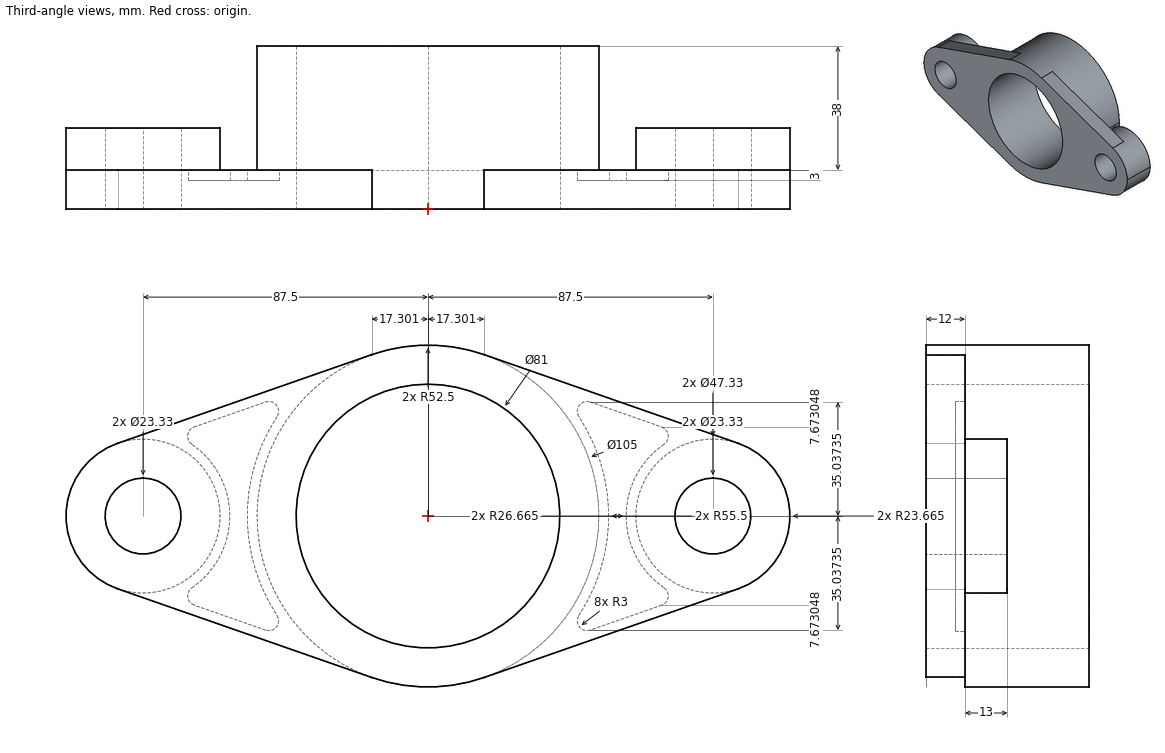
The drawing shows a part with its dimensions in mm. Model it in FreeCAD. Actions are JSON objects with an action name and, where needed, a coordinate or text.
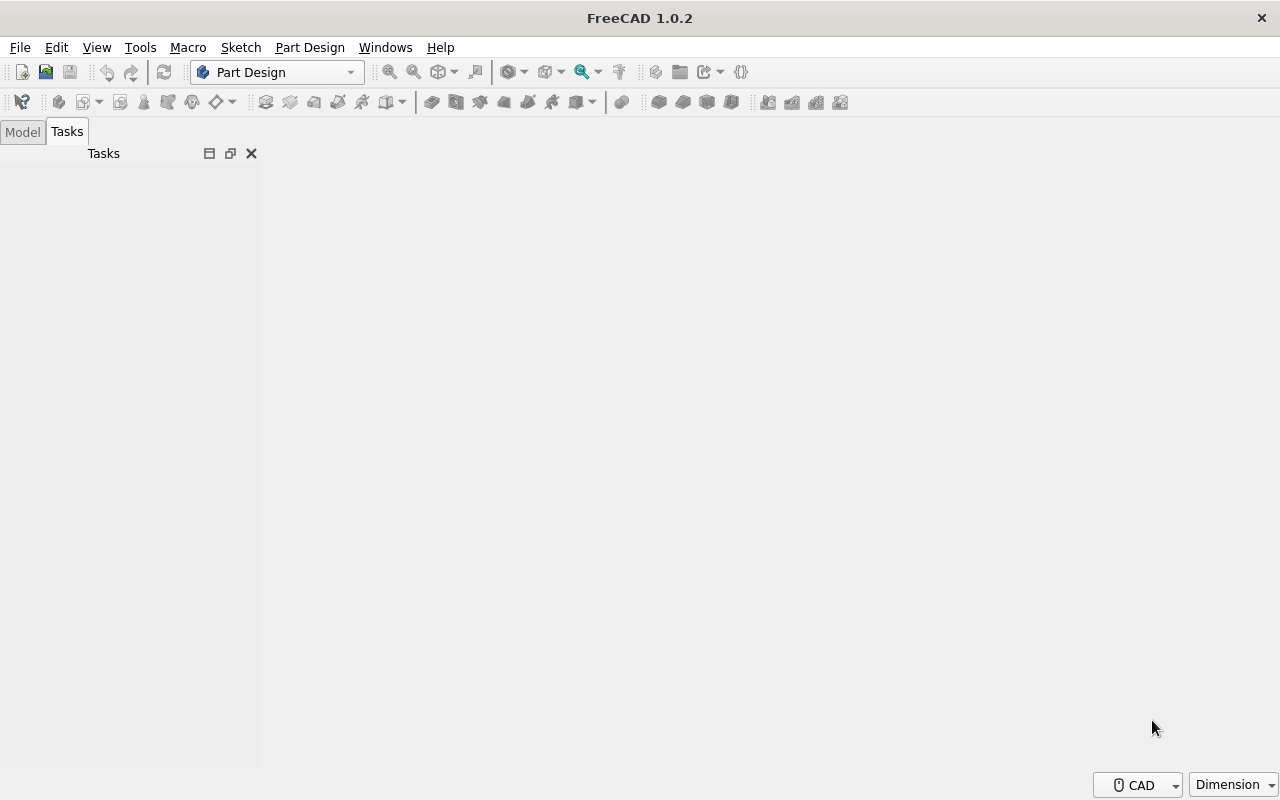
{"action": "left_click", "coordinate": [22, 72]}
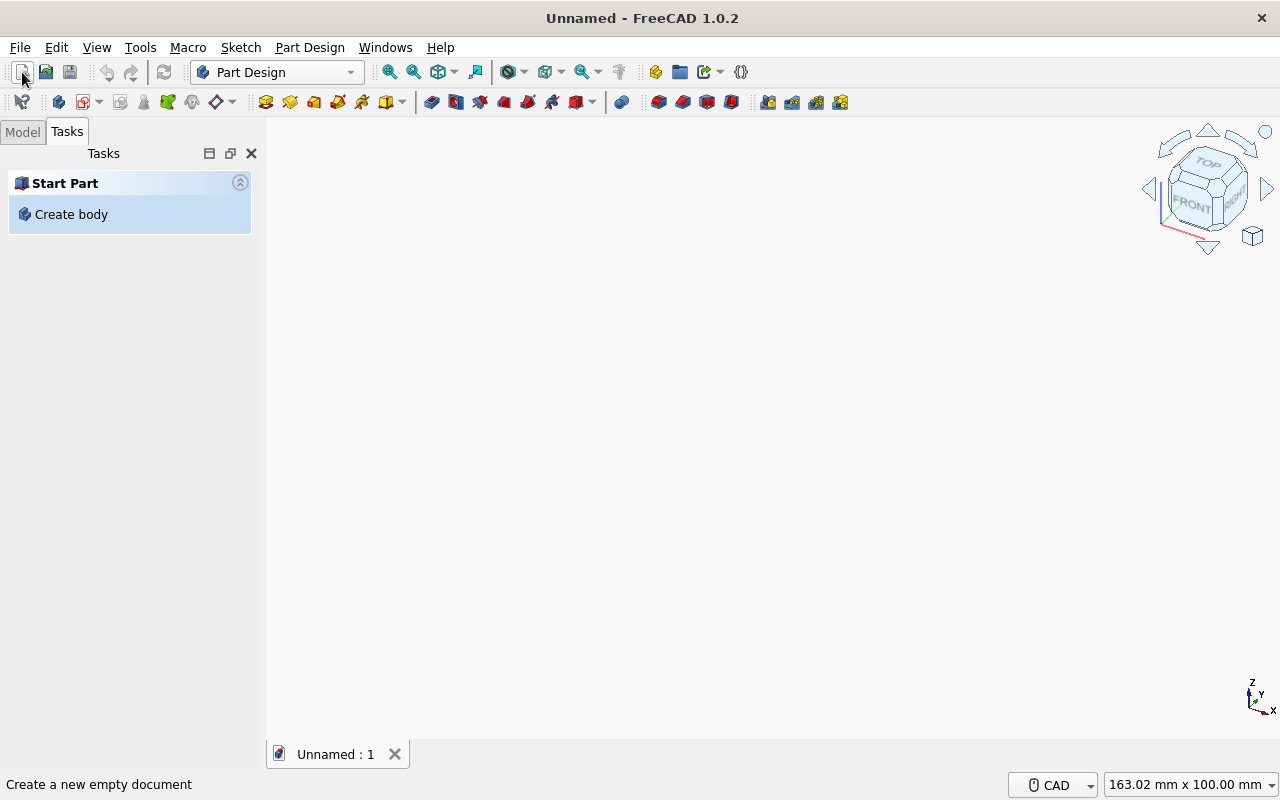
{"action": "left_click", "coordinate": [84, 102]}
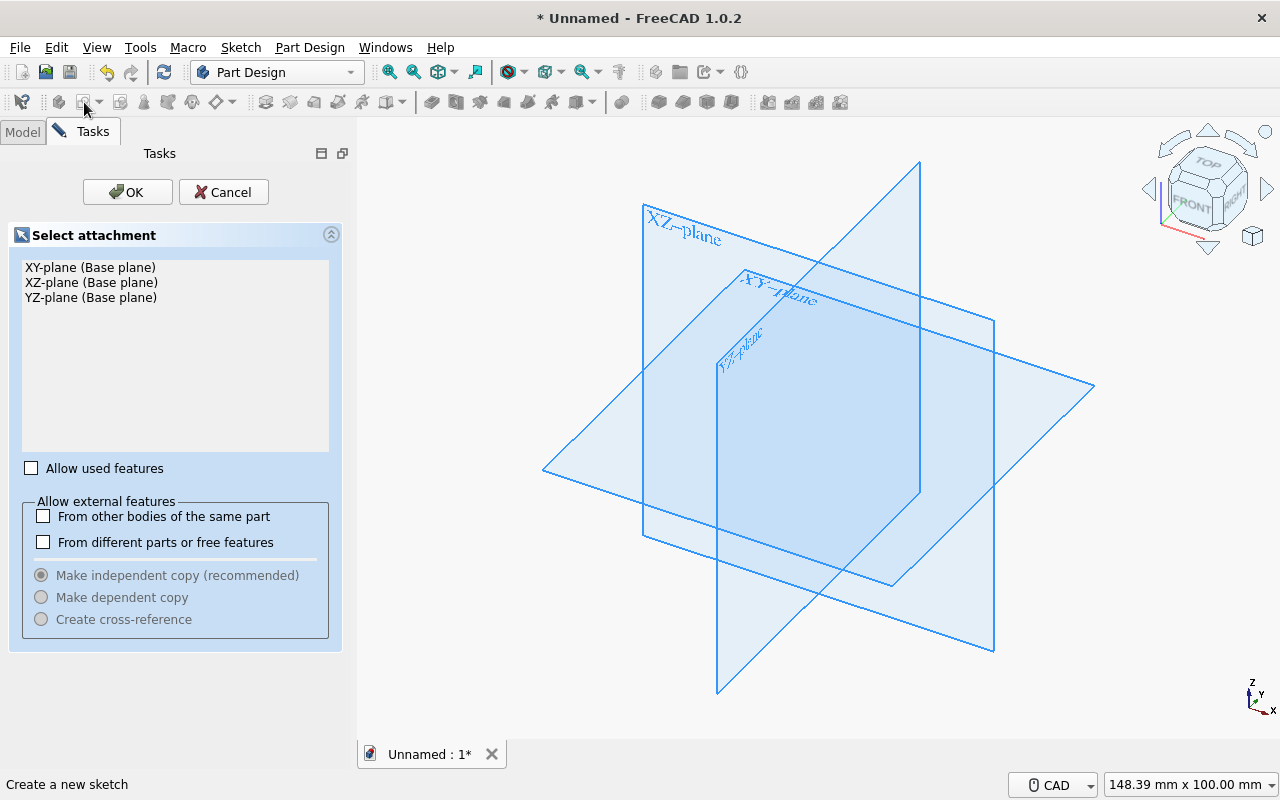
{"action": "left_click", "coordinate": [82, 282]}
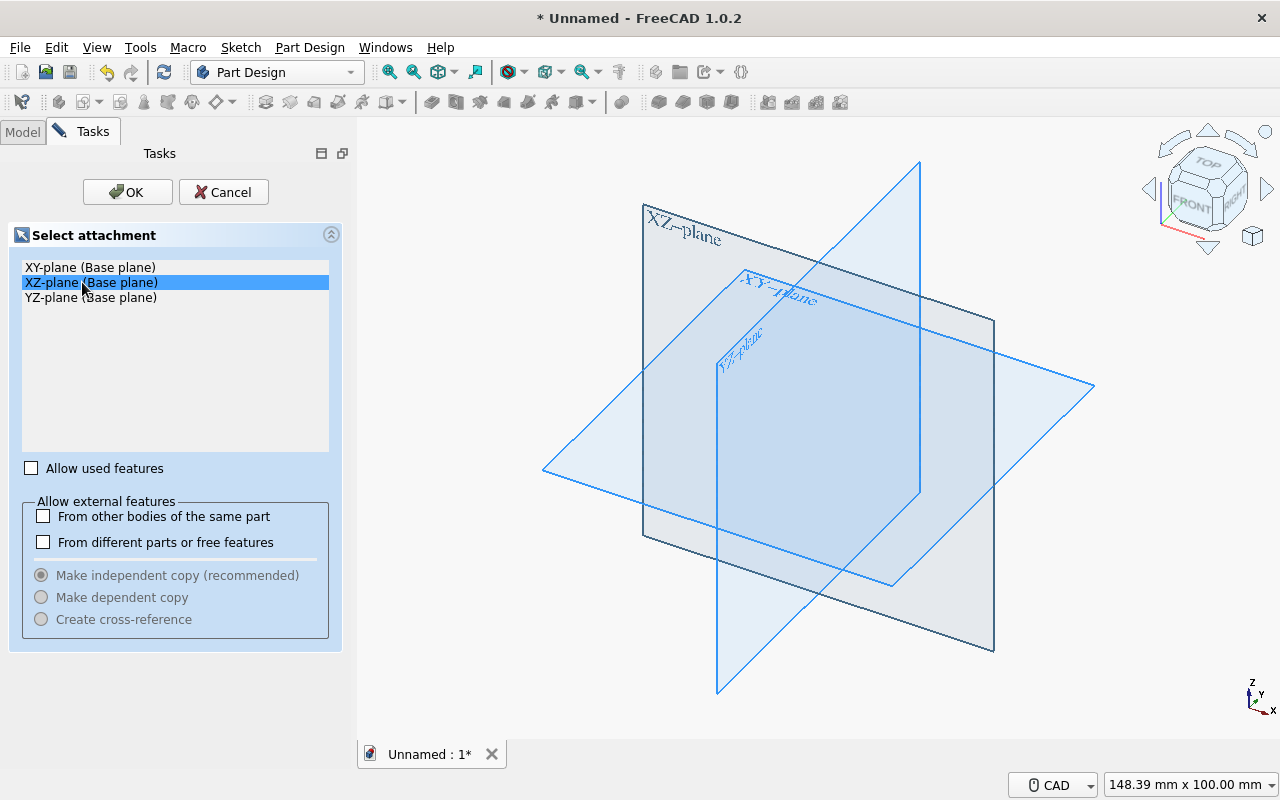
{"action": "left_click", "coordinate": [128, 192]}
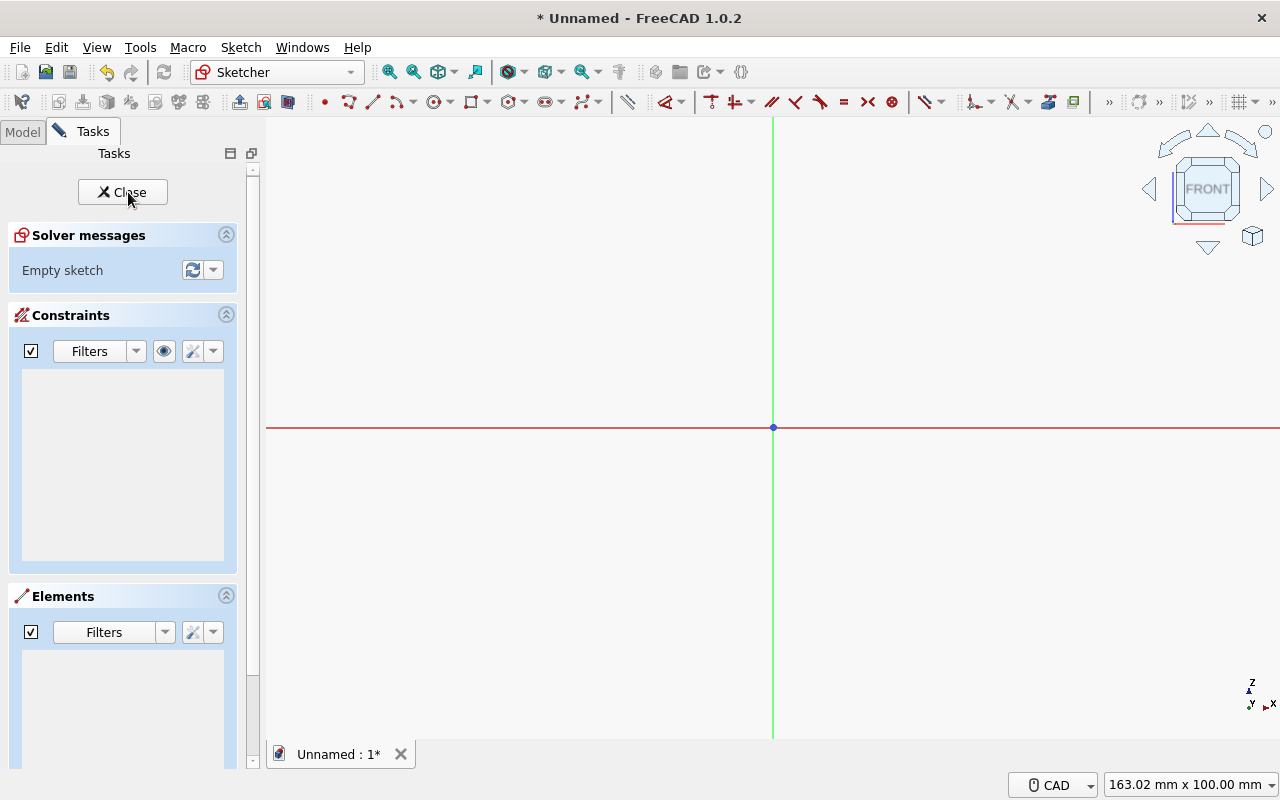
{"action": "scroll", "coordinate": [649, 428], "scroll_direction": "down", "scroll_amount": 4}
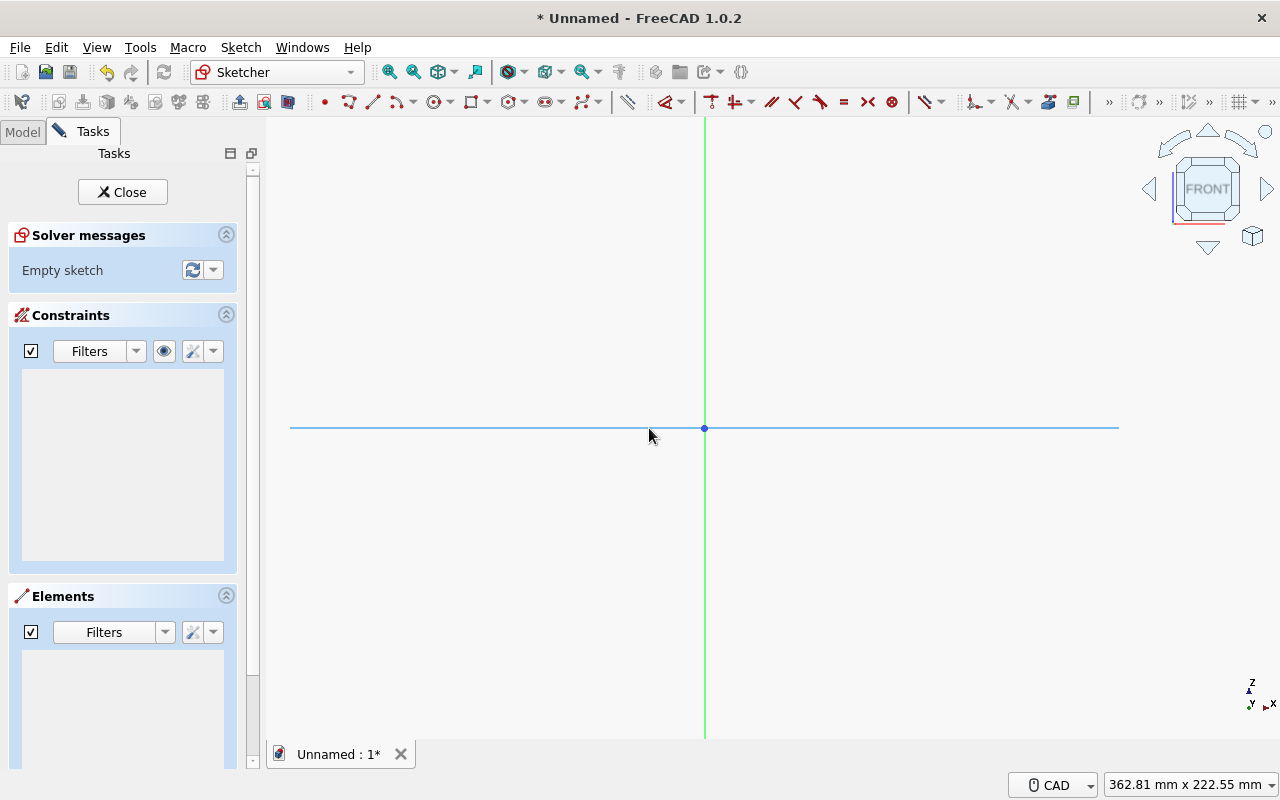
{"action": "left_click", "coordinate": [374, 102]}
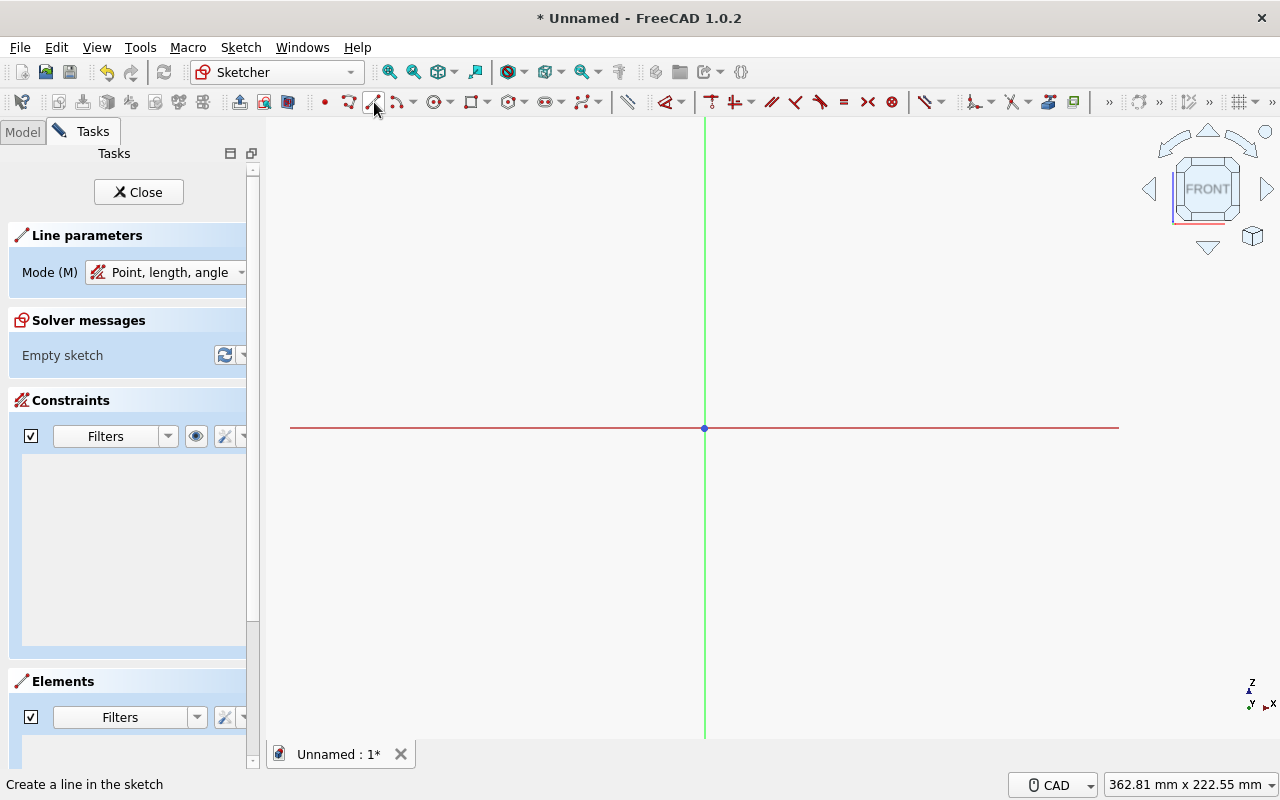
{"action": "left_click", "coordinate": [439, 366]}
{"action": "left_click", "coordinate": [657, 290]}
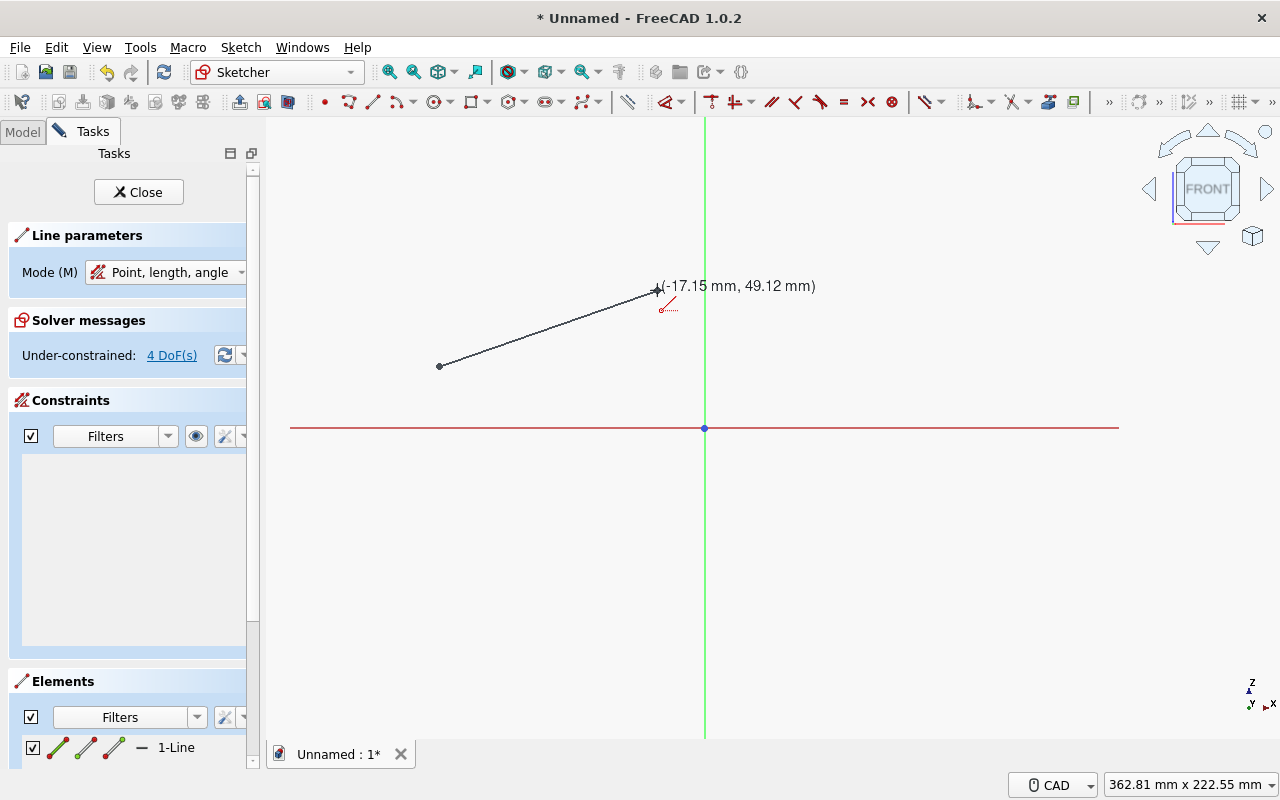
{"action": "left_click", "coordinate": [753, 290]}
{"action": "left_click", "coordinate": [971, 366]}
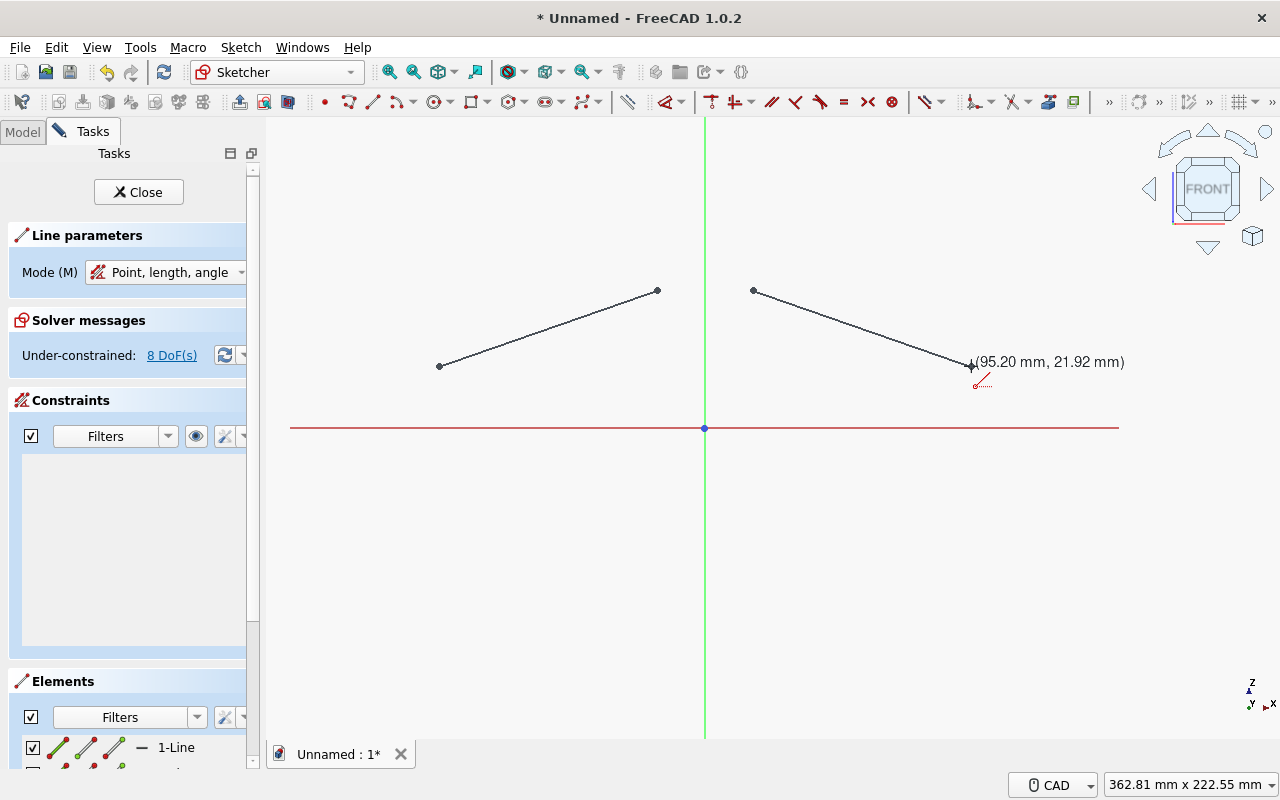
{"action": "left_click", "coordinate": [971, 491]}
{"action": "left_click", "coordinate": [753, 567]}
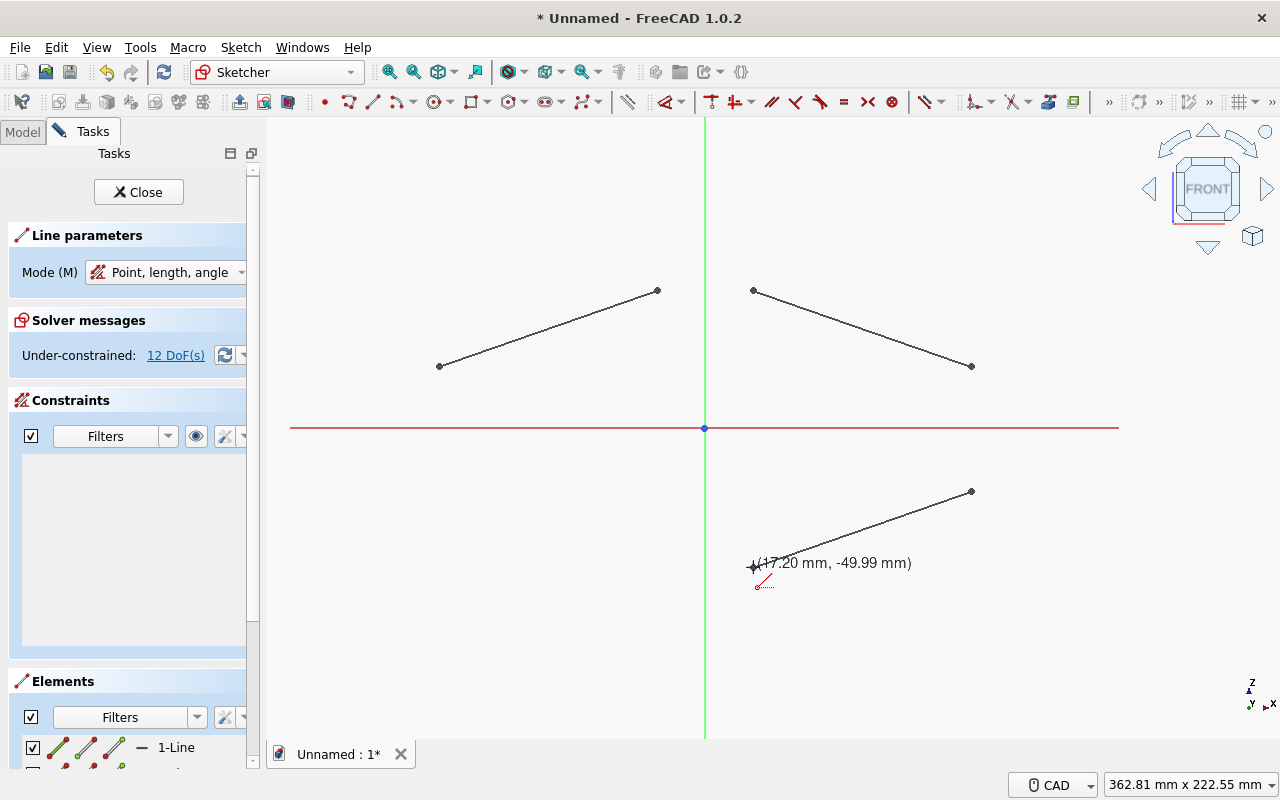
{"action": "left_click", "coordinate": [657, 567]}
{"action": "left_click", "coordinate": [439, 491]}